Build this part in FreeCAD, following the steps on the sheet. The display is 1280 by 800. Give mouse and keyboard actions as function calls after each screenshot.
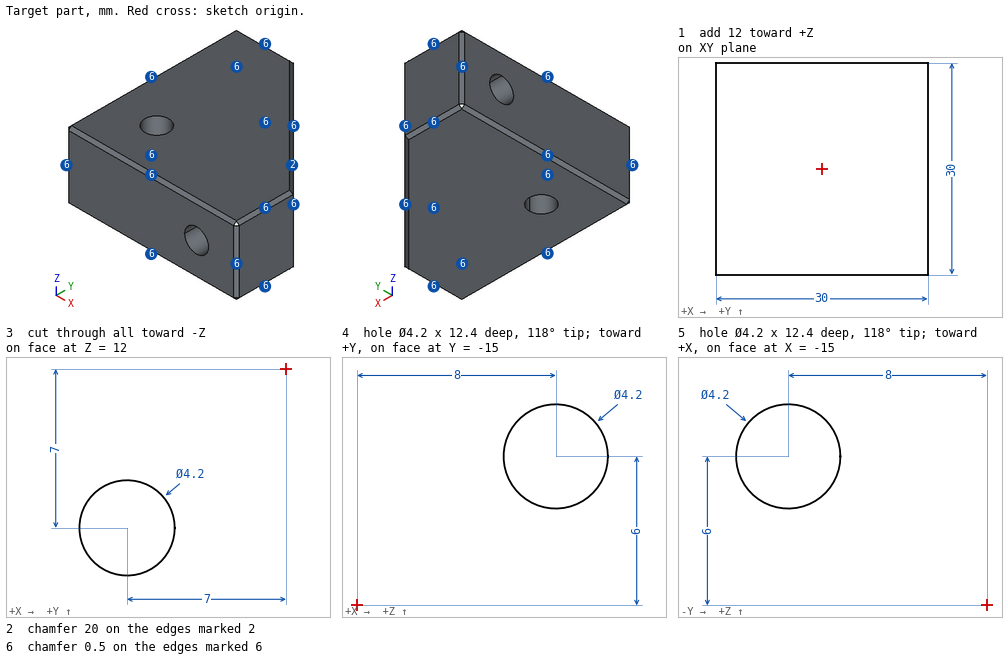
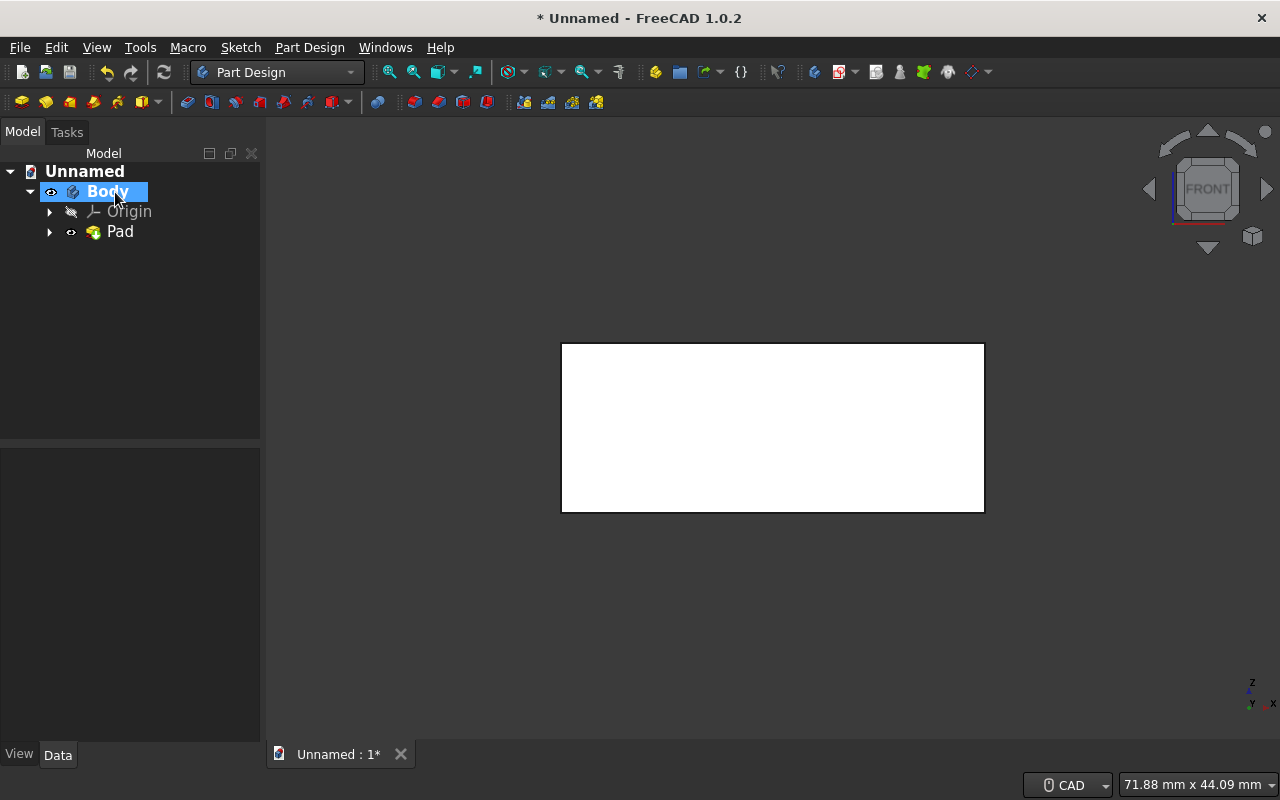
key(v)
key(f)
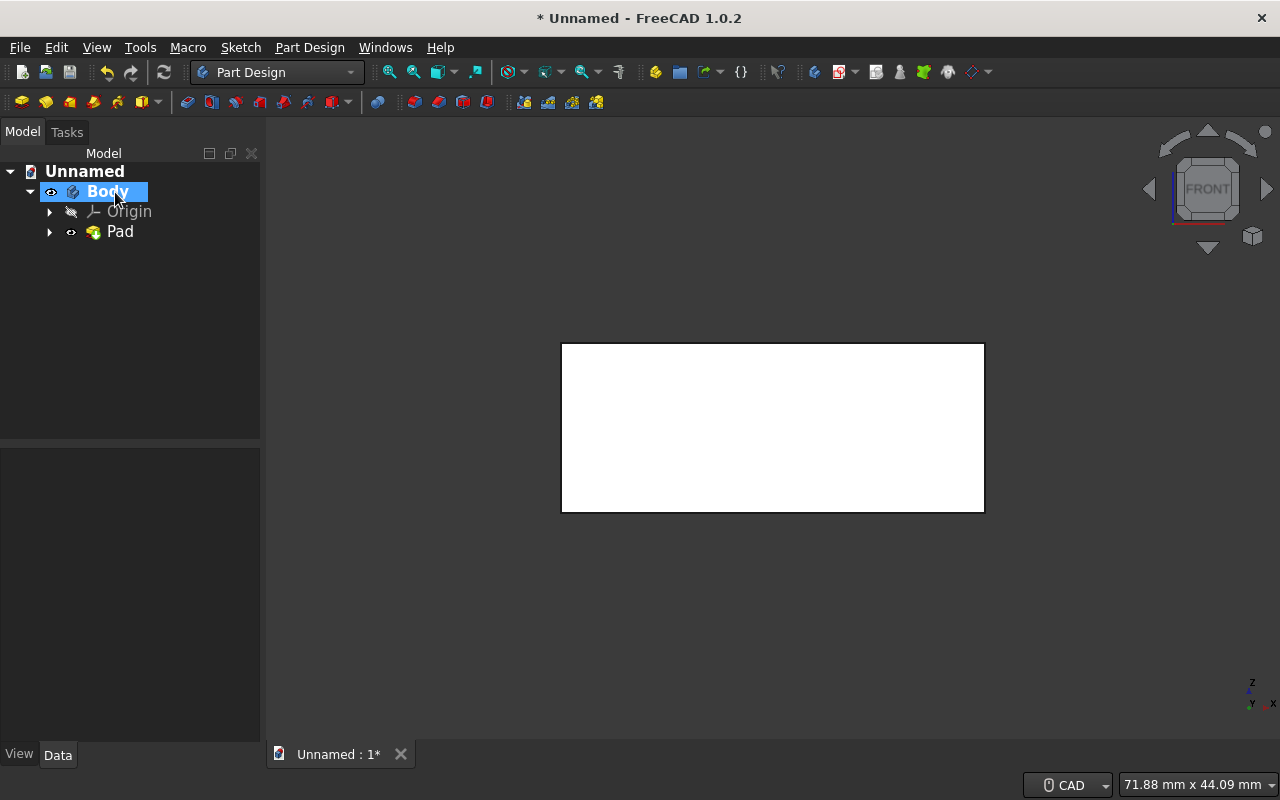
key(3)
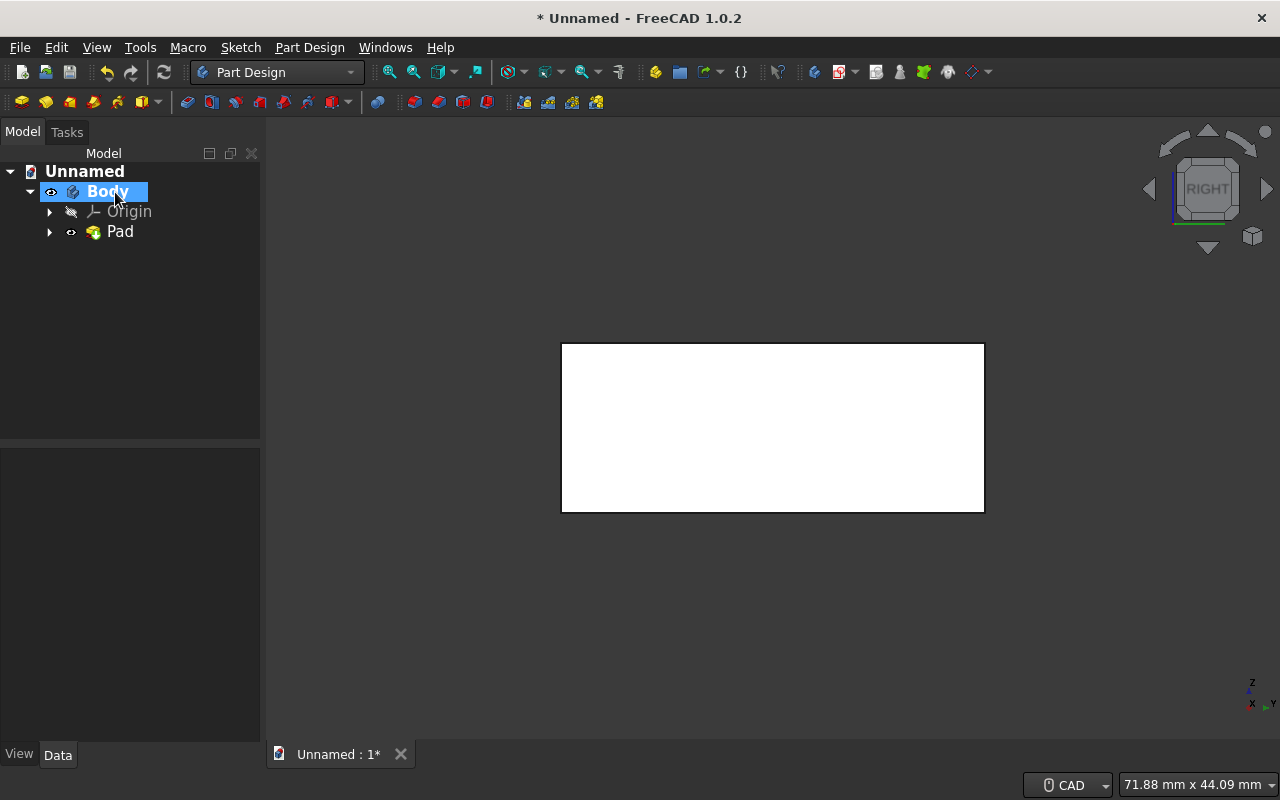
key(v)
key(f)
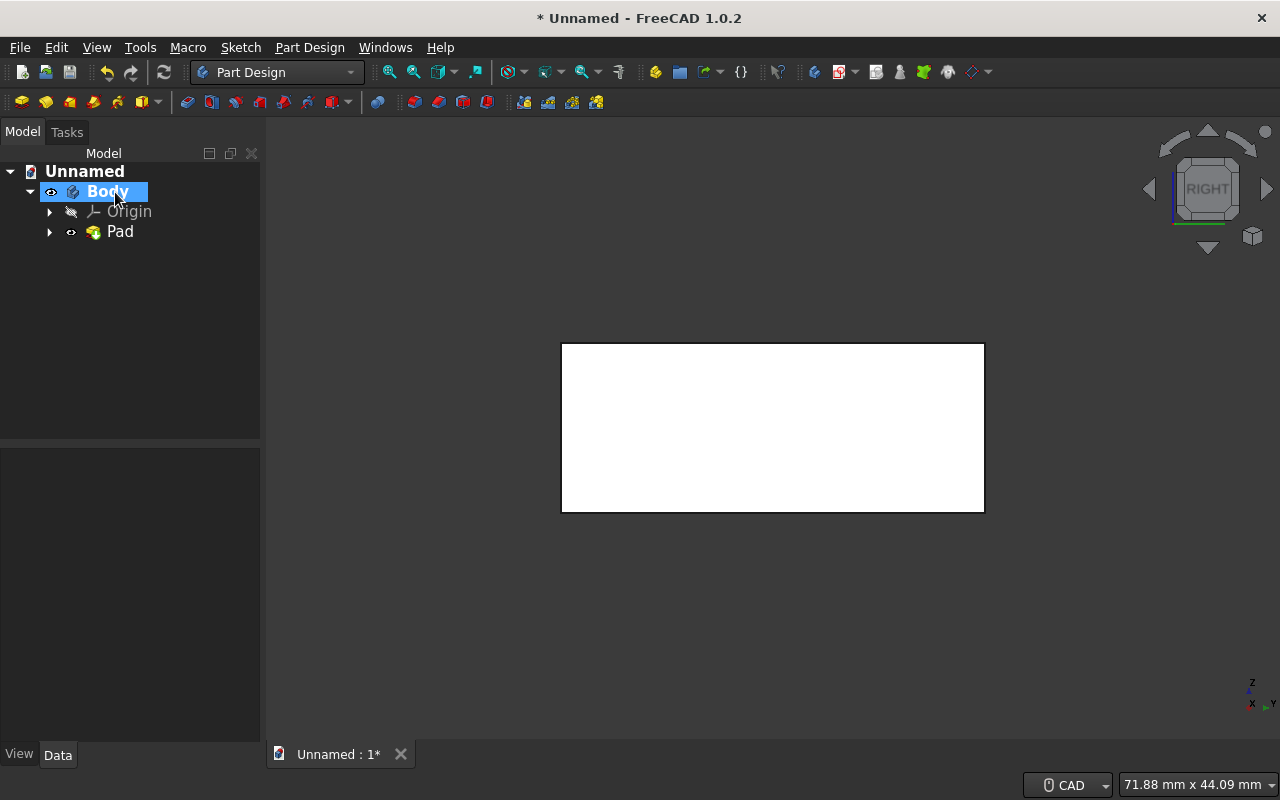
click(985, 427)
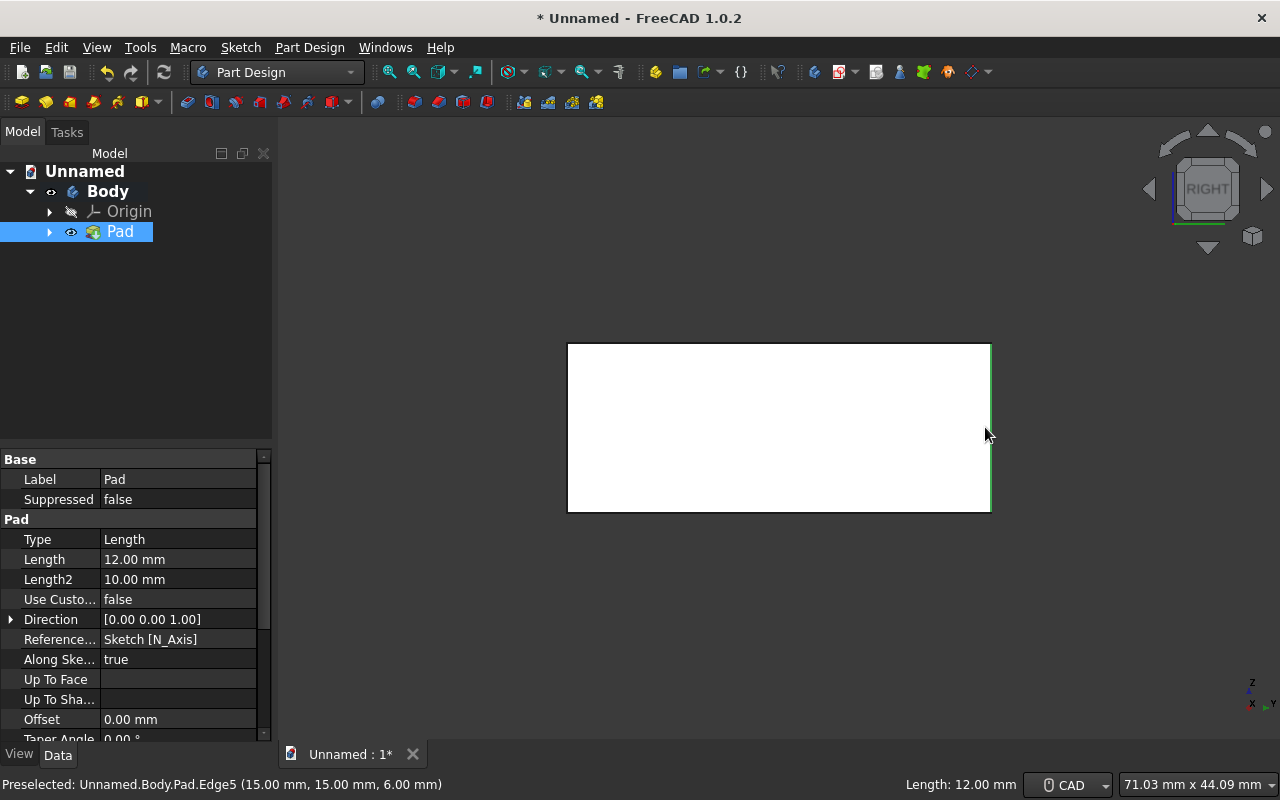
click(440, 102)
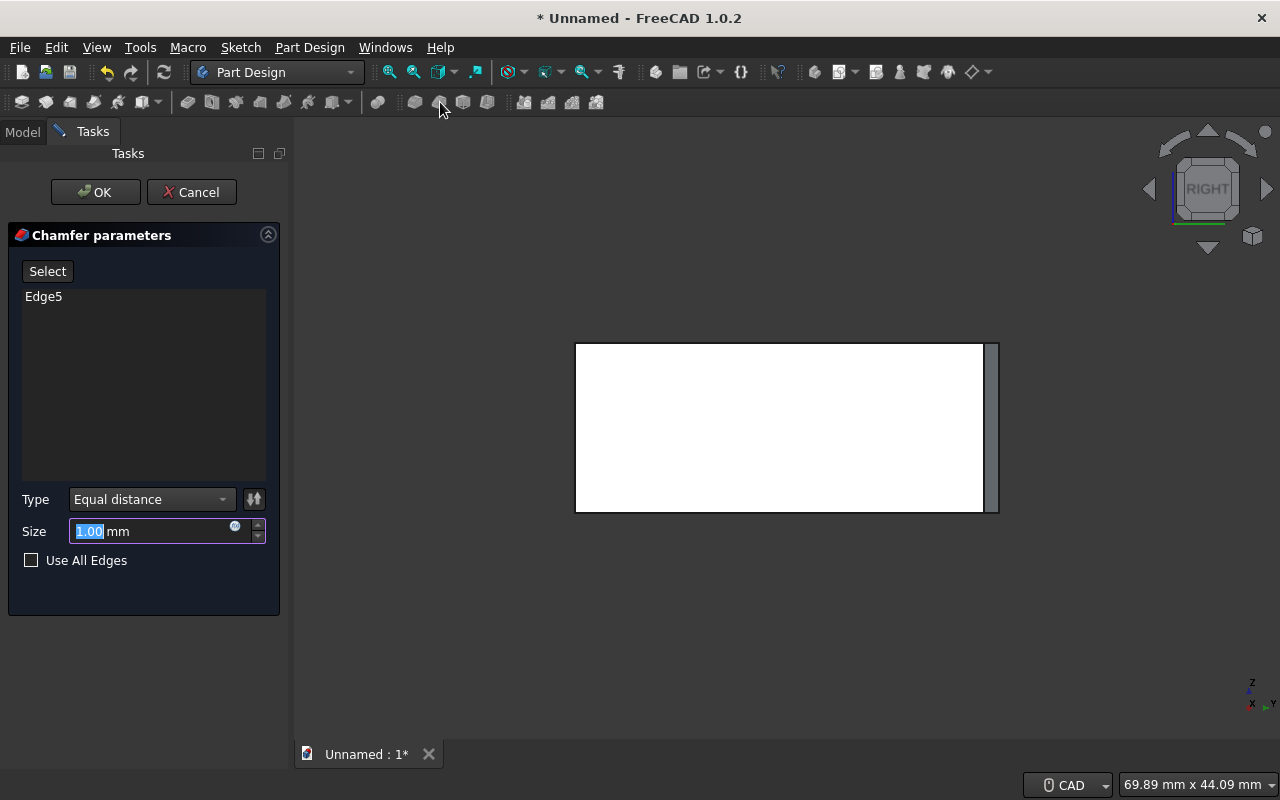
text(20)
key(Tab)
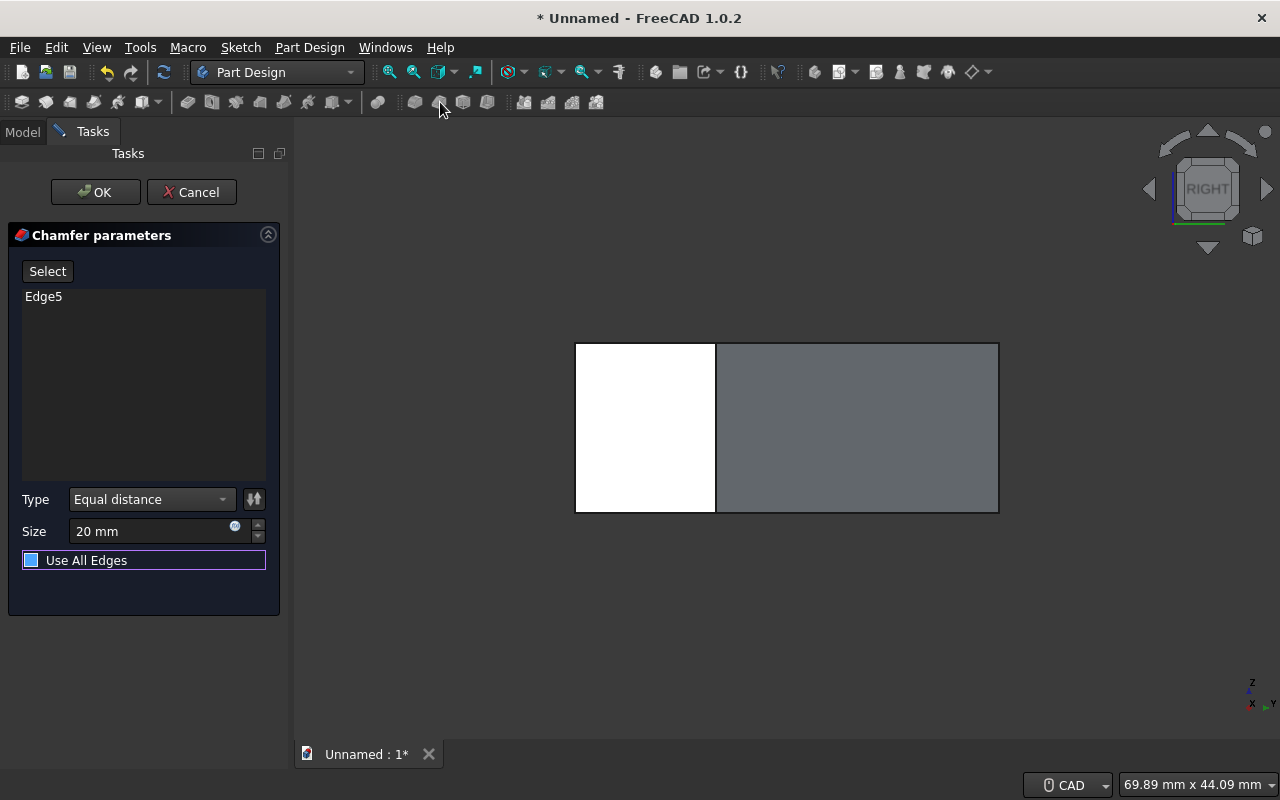
click(96, 192)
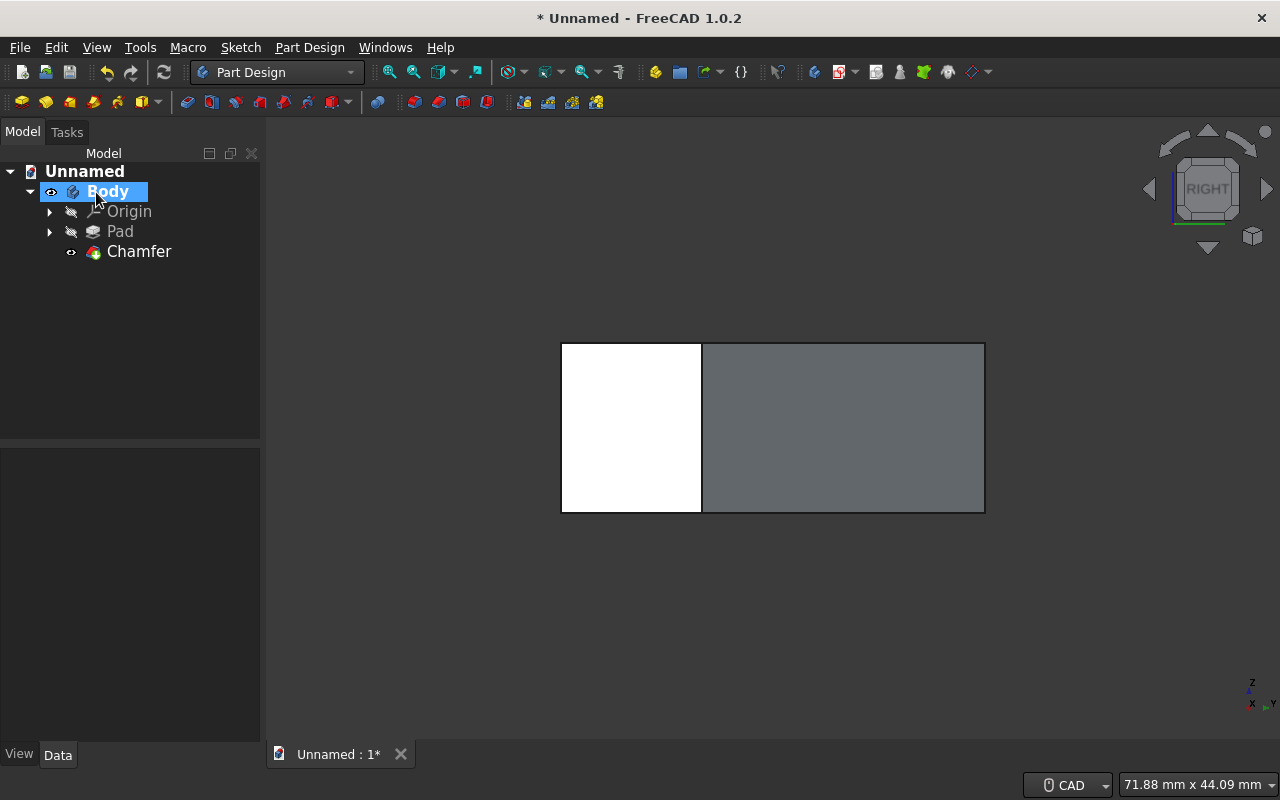
key(v)
key(f)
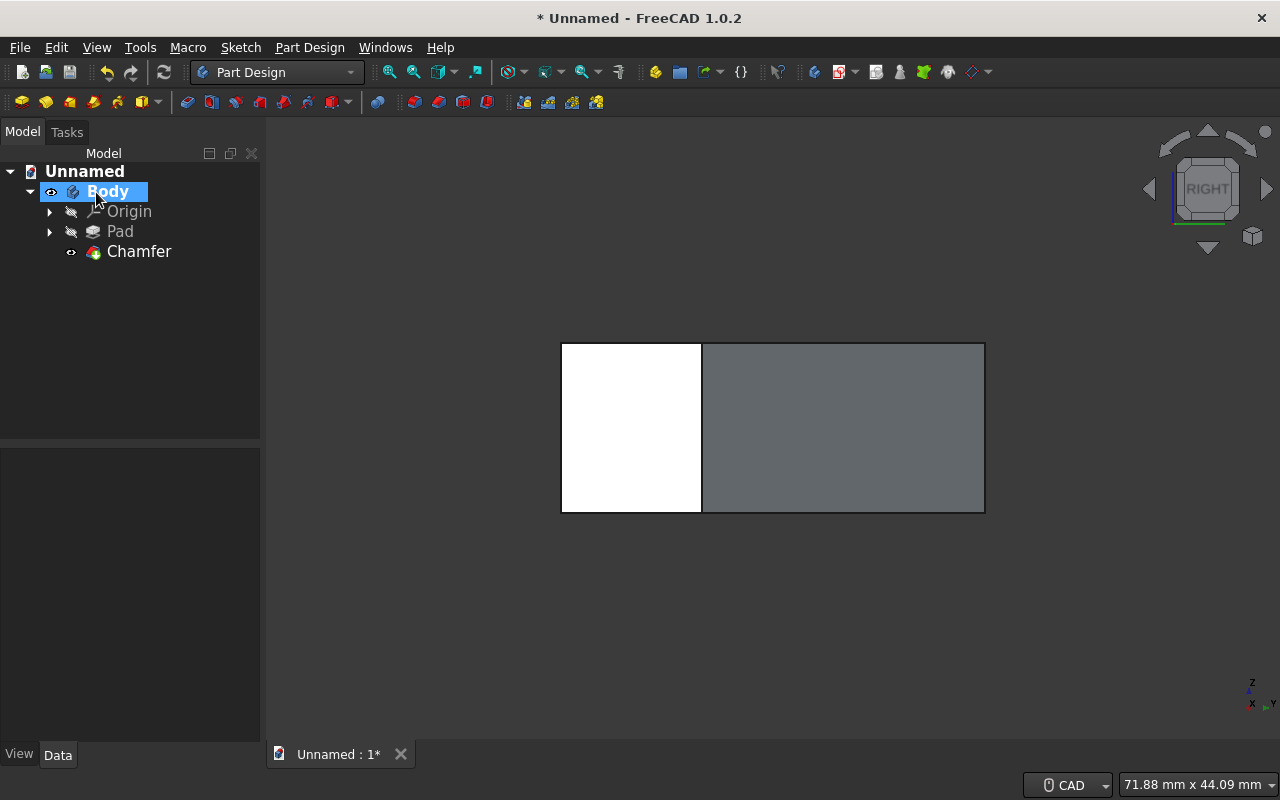
key(0)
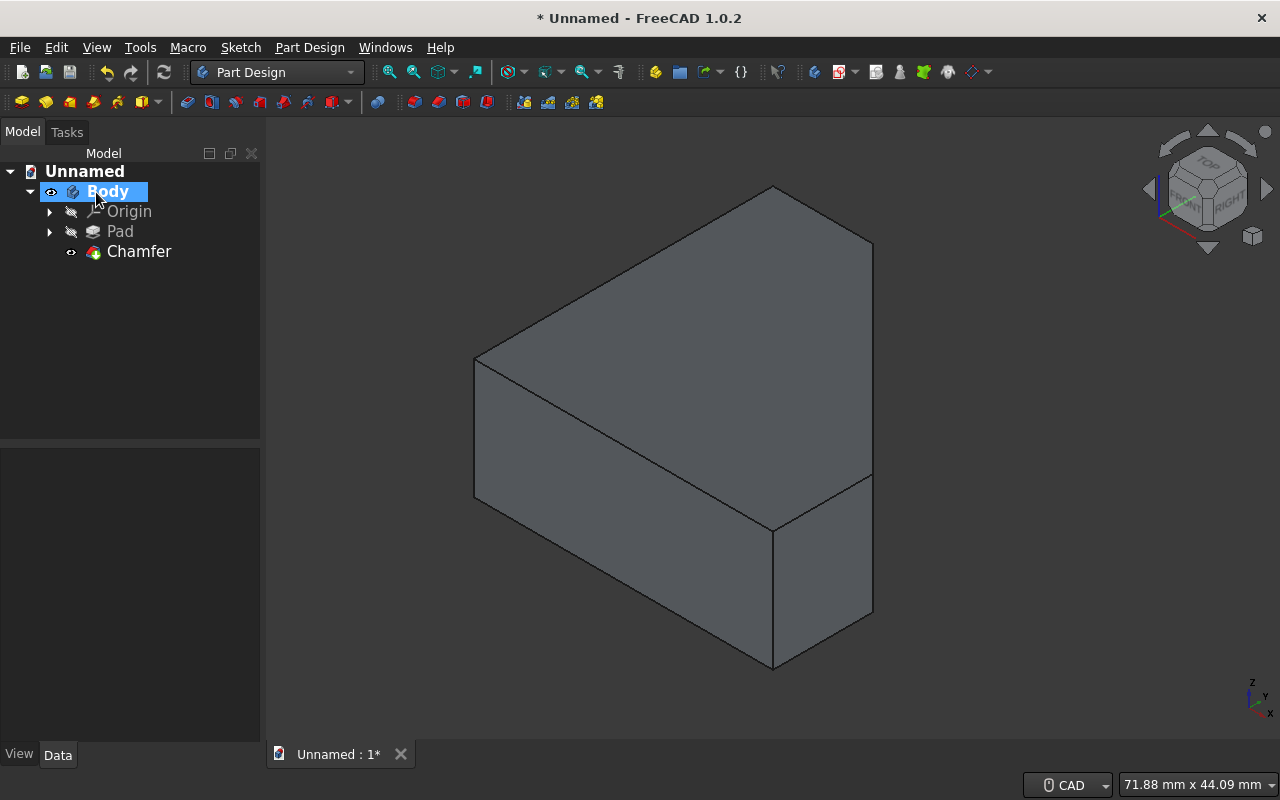
click(687, 358)